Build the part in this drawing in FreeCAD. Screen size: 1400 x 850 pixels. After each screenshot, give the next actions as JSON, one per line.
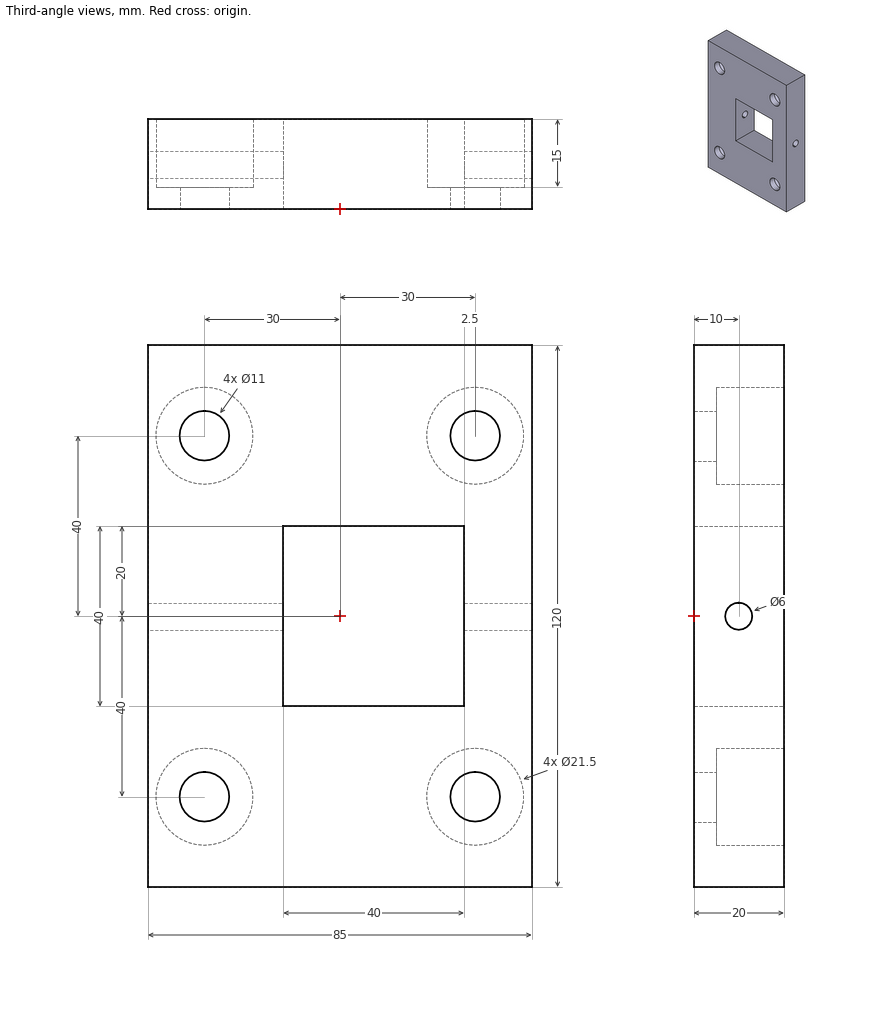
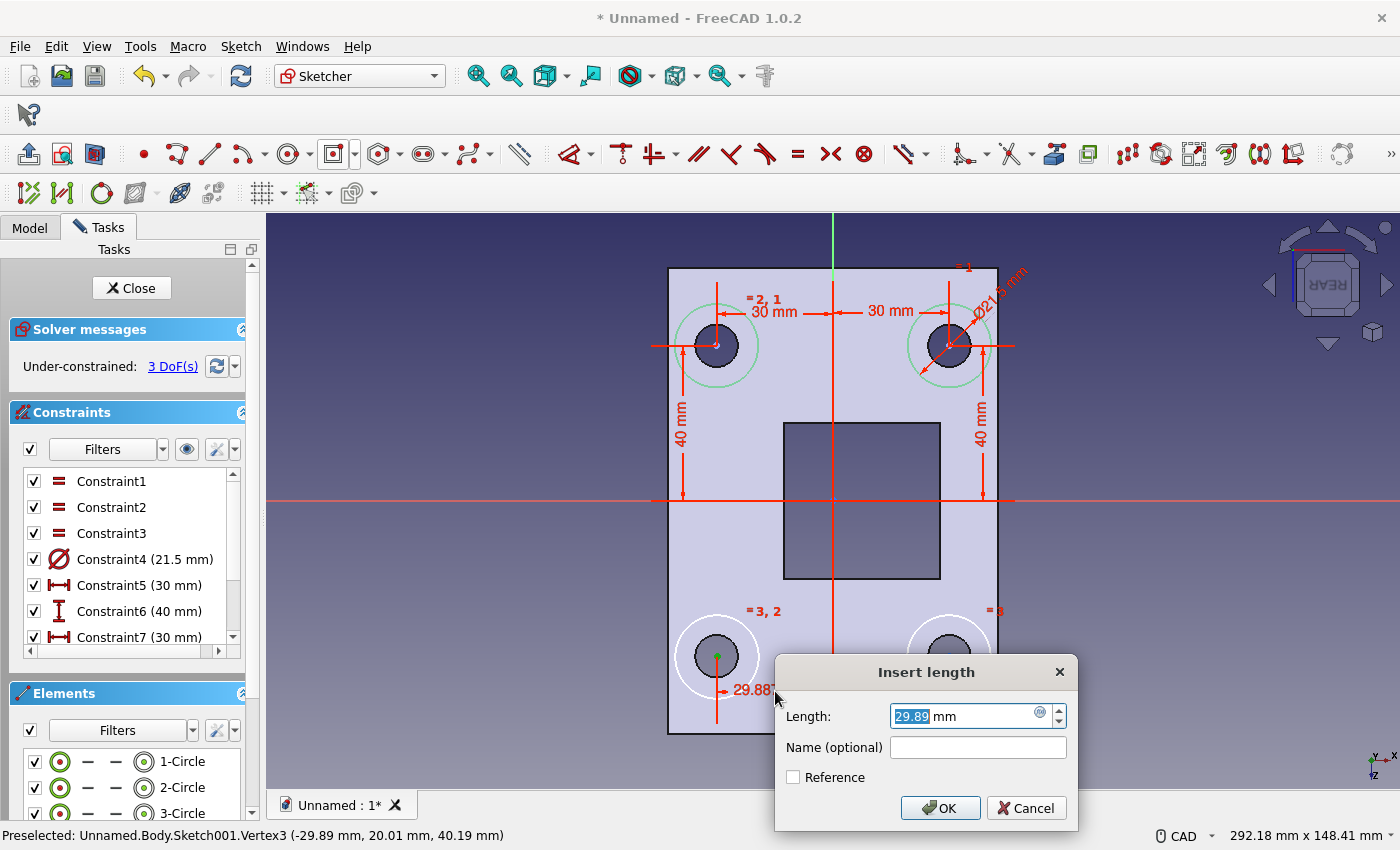
{"action": "type", "text": "30"}
{"action": "key", "text": "Return"}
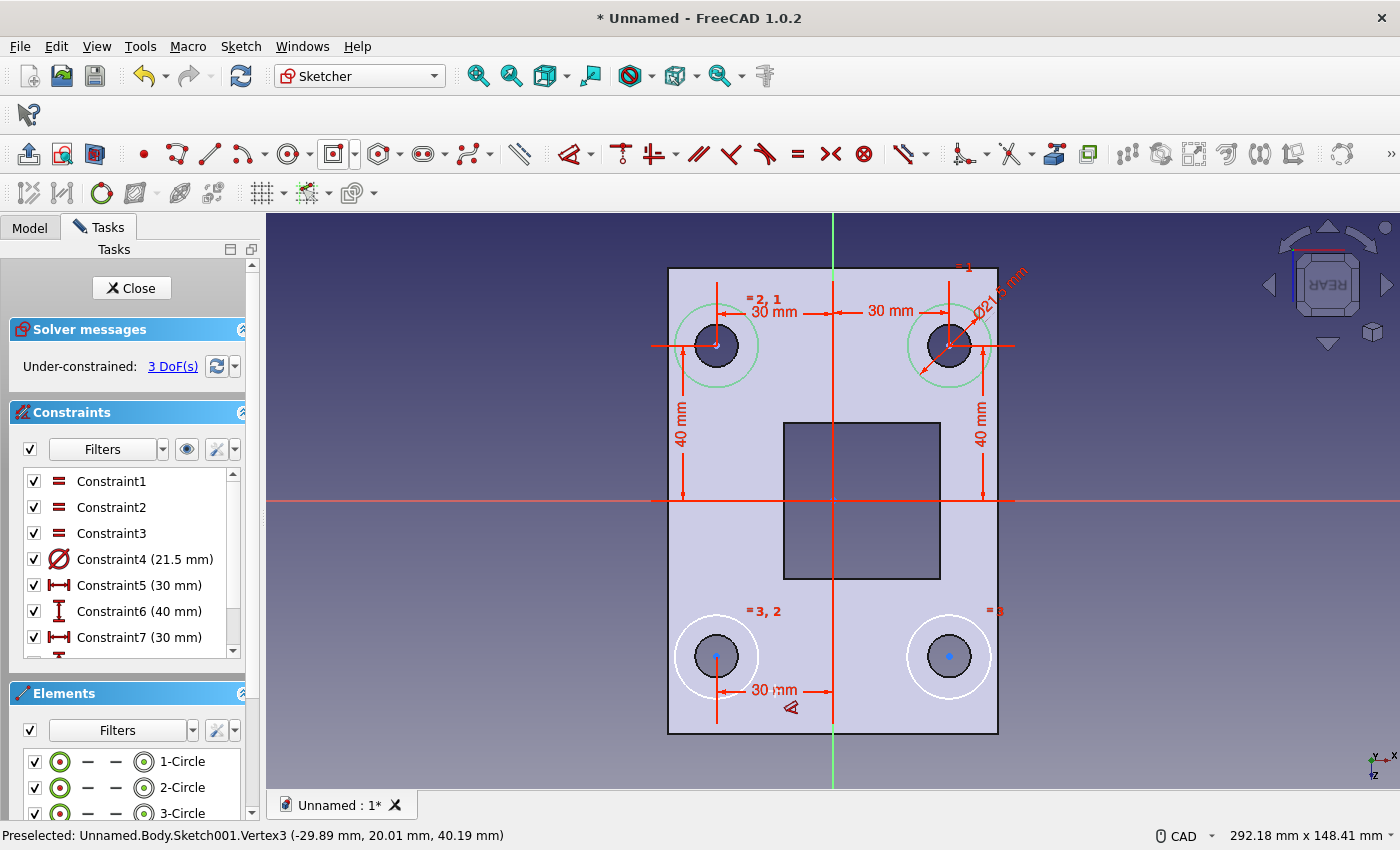
{"action": "left_click", "coordinate": [717, 657]}
{"action": "left_click", "coordinate": [683, 579]}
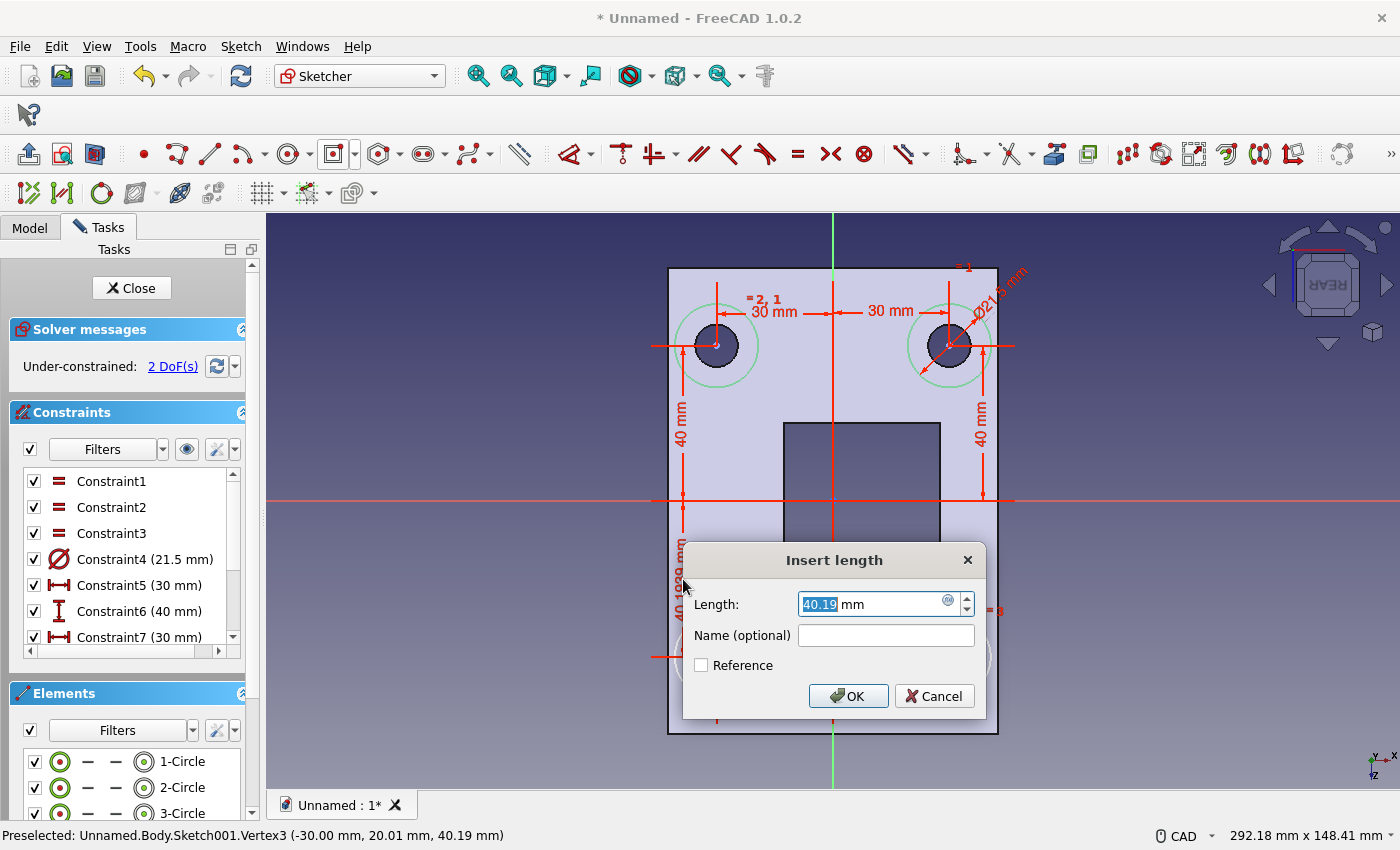
{"action": "type", "text": "40"}
{"action": "key", "text": "Return"}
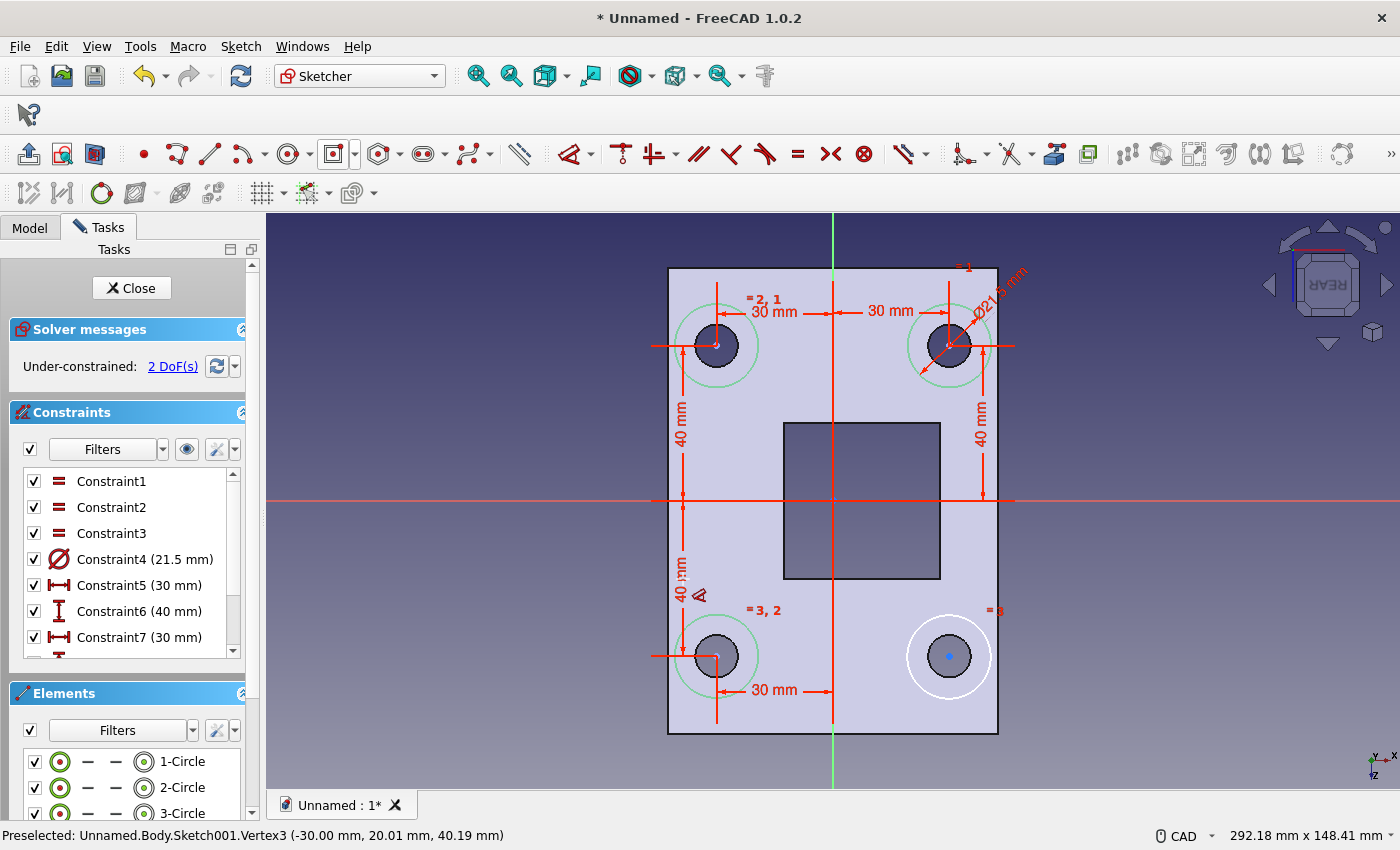
{"action": "left_click", "coordinate": [949, 657]}
{"action": "left_click", "coordinate": [891, 691]}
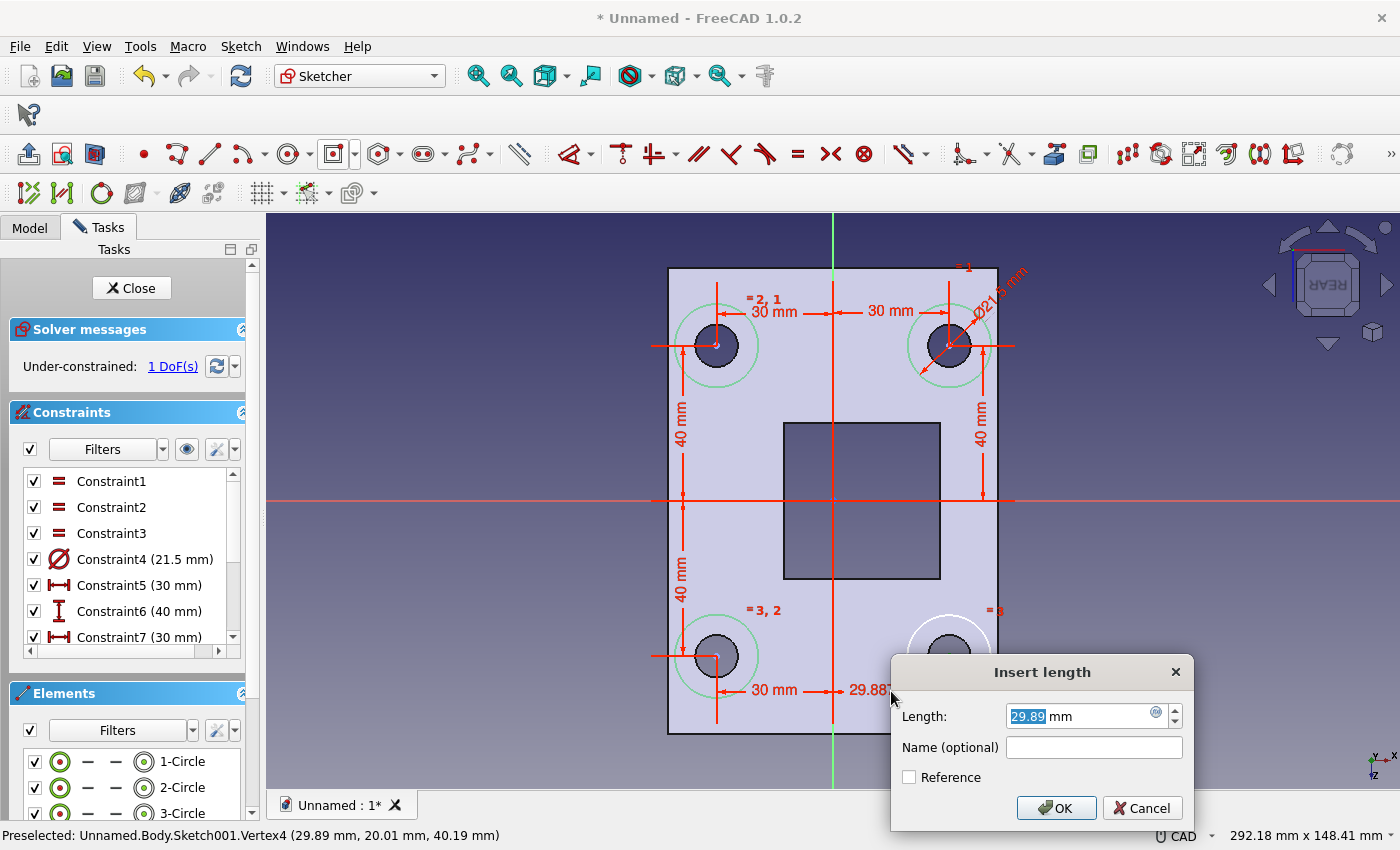
{"action": "type", "text": "30"}
{"action": "key", "text": "Return"}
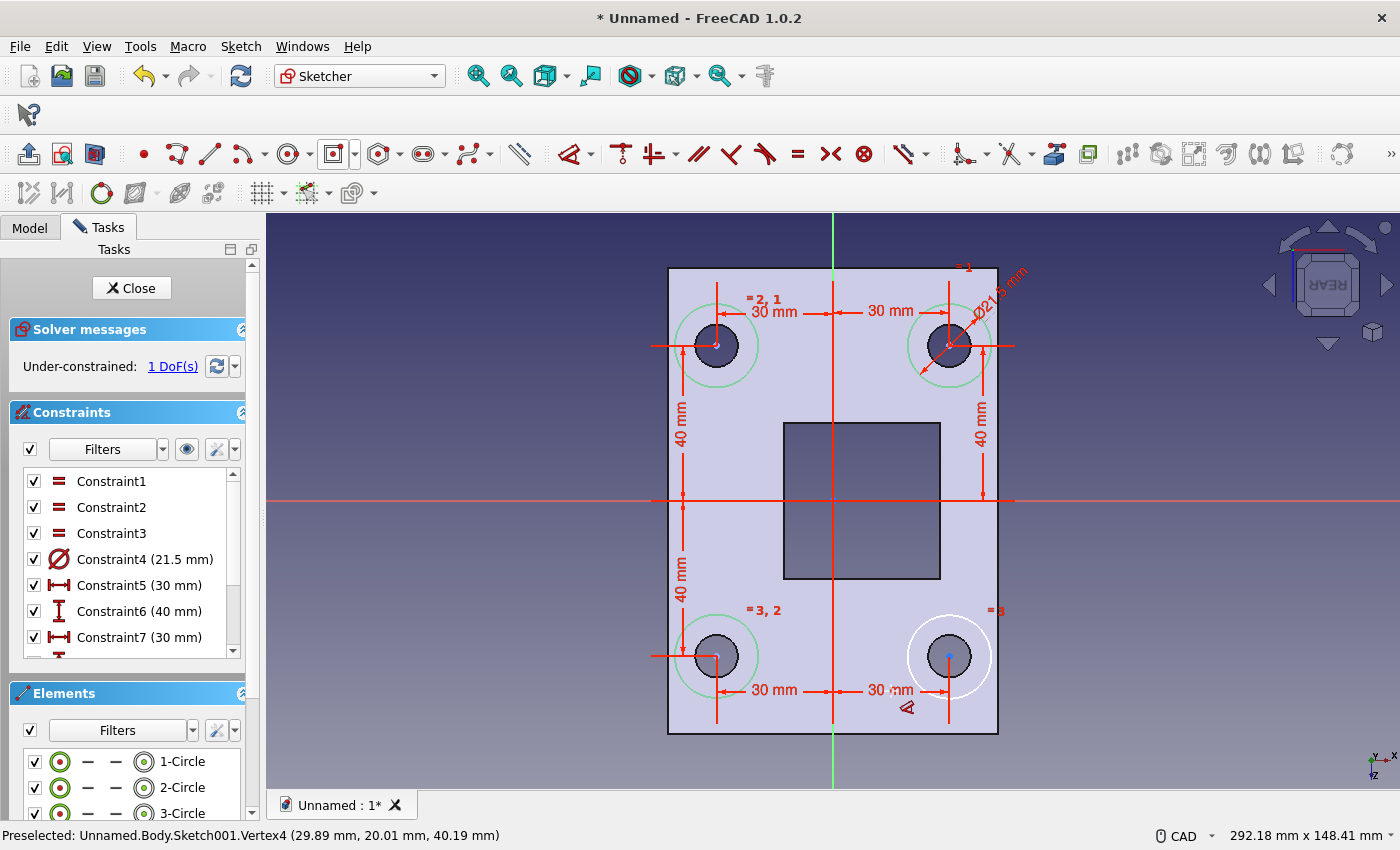
{"action": "left_click", "coordinate": [949, 657]}
{"action": "left_click", "coordinate": [983, 579]}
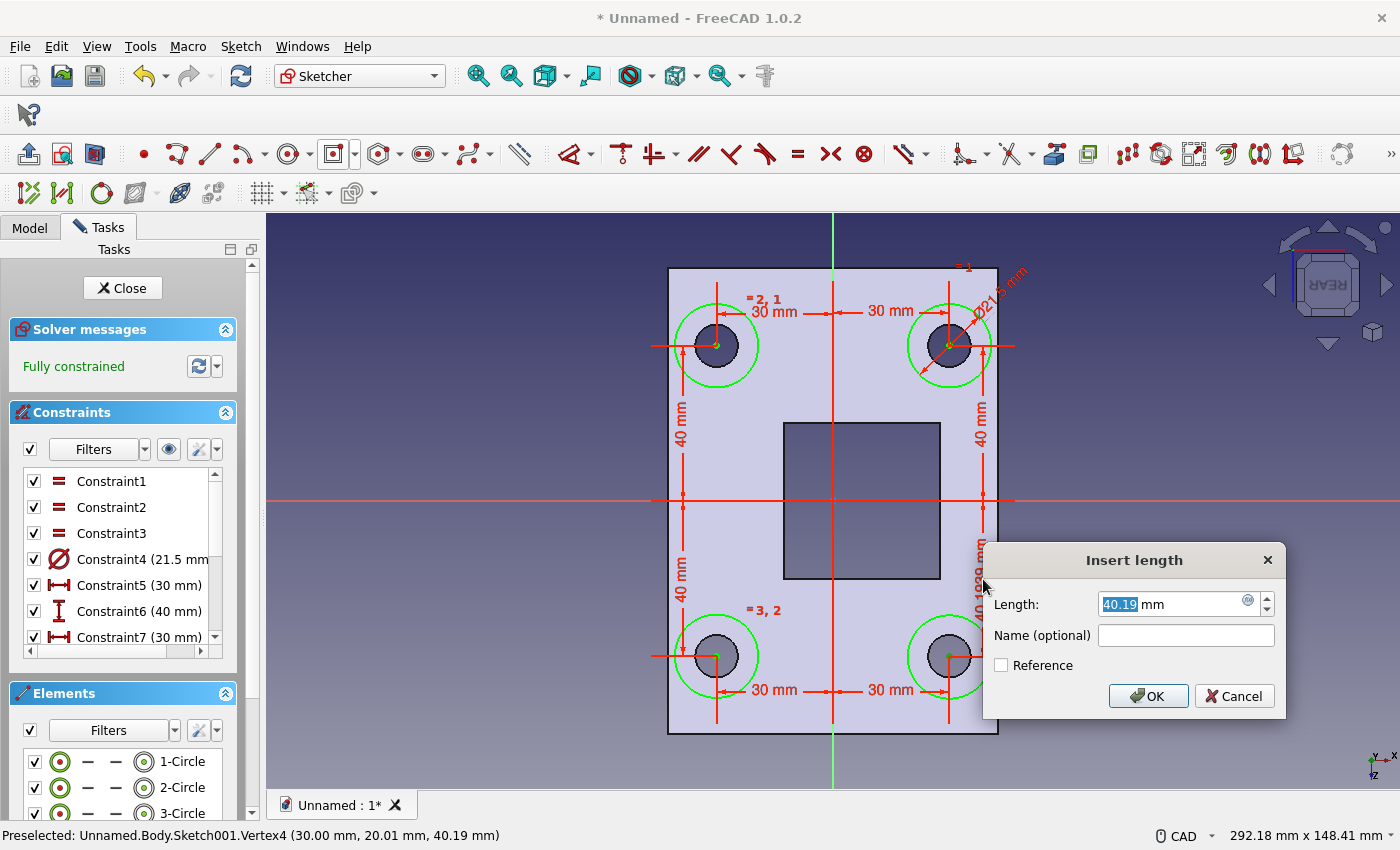
{"action": "type", "text": "40"}
{"action": "key", "text": "Return"}
{"action": "key", "text": "Escape"}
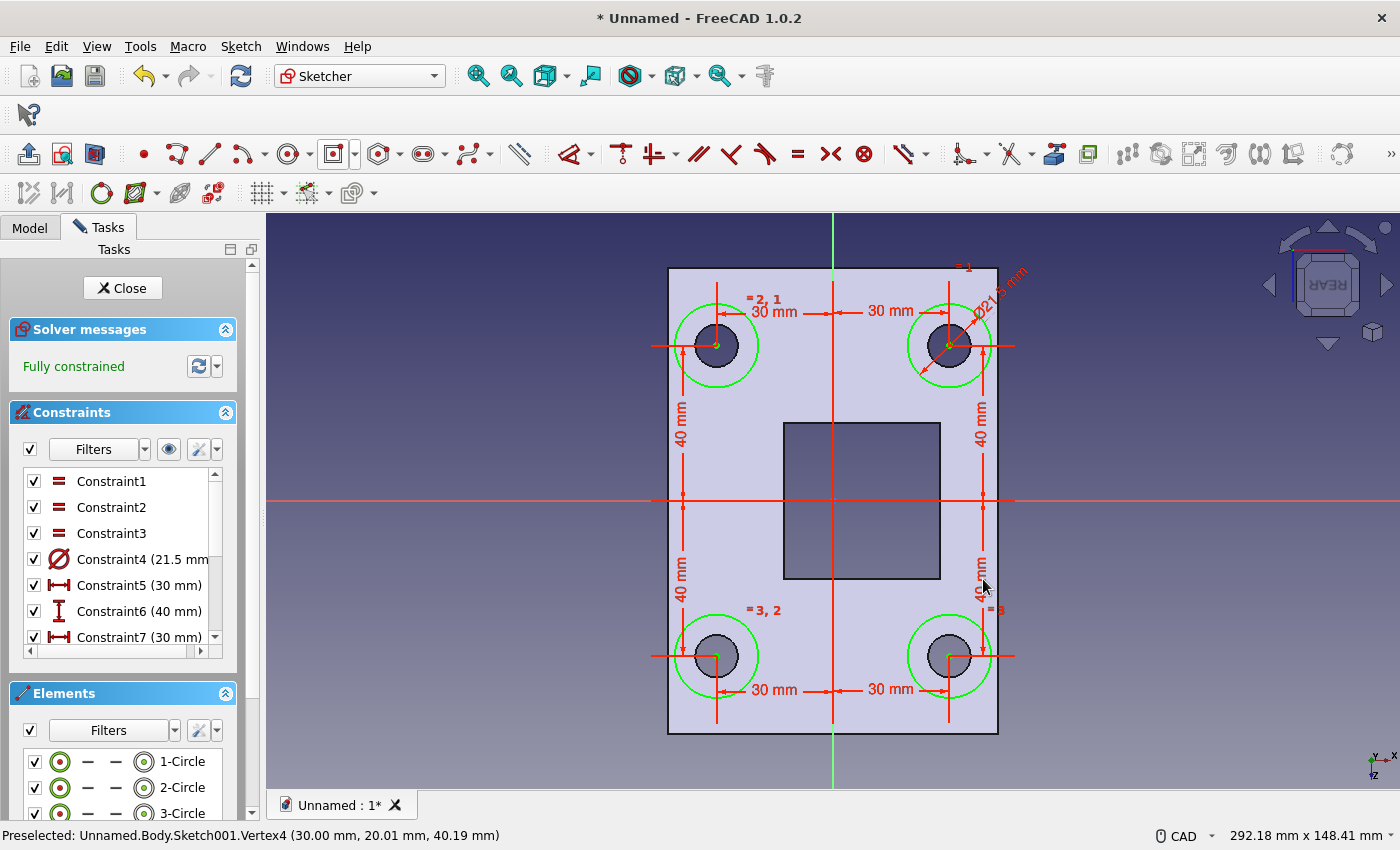
{"action": "left_click", "coordinate": [123, 288]}